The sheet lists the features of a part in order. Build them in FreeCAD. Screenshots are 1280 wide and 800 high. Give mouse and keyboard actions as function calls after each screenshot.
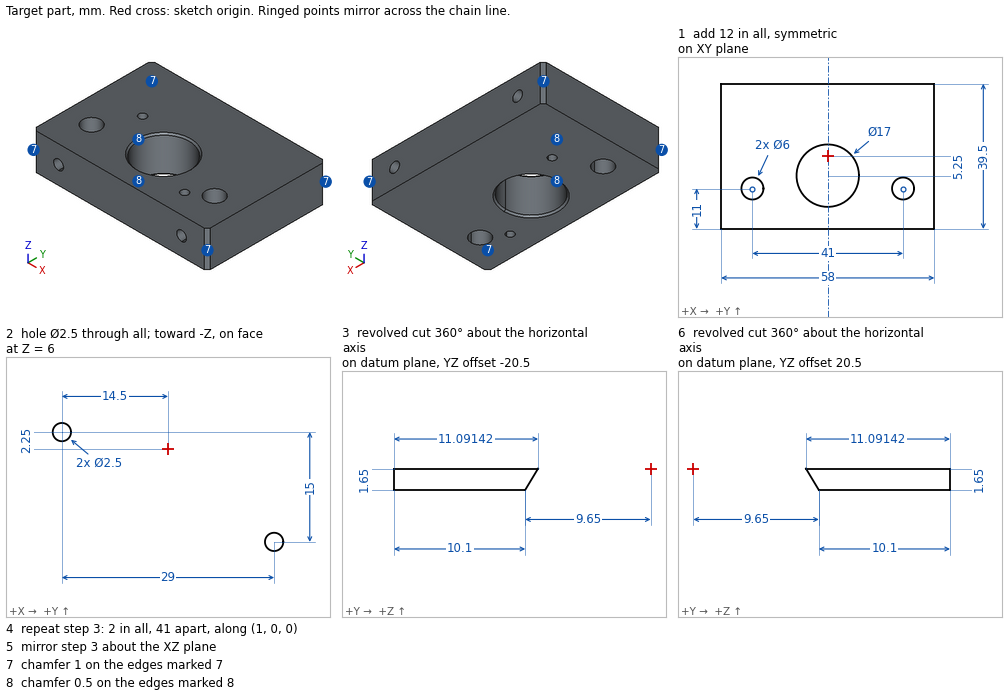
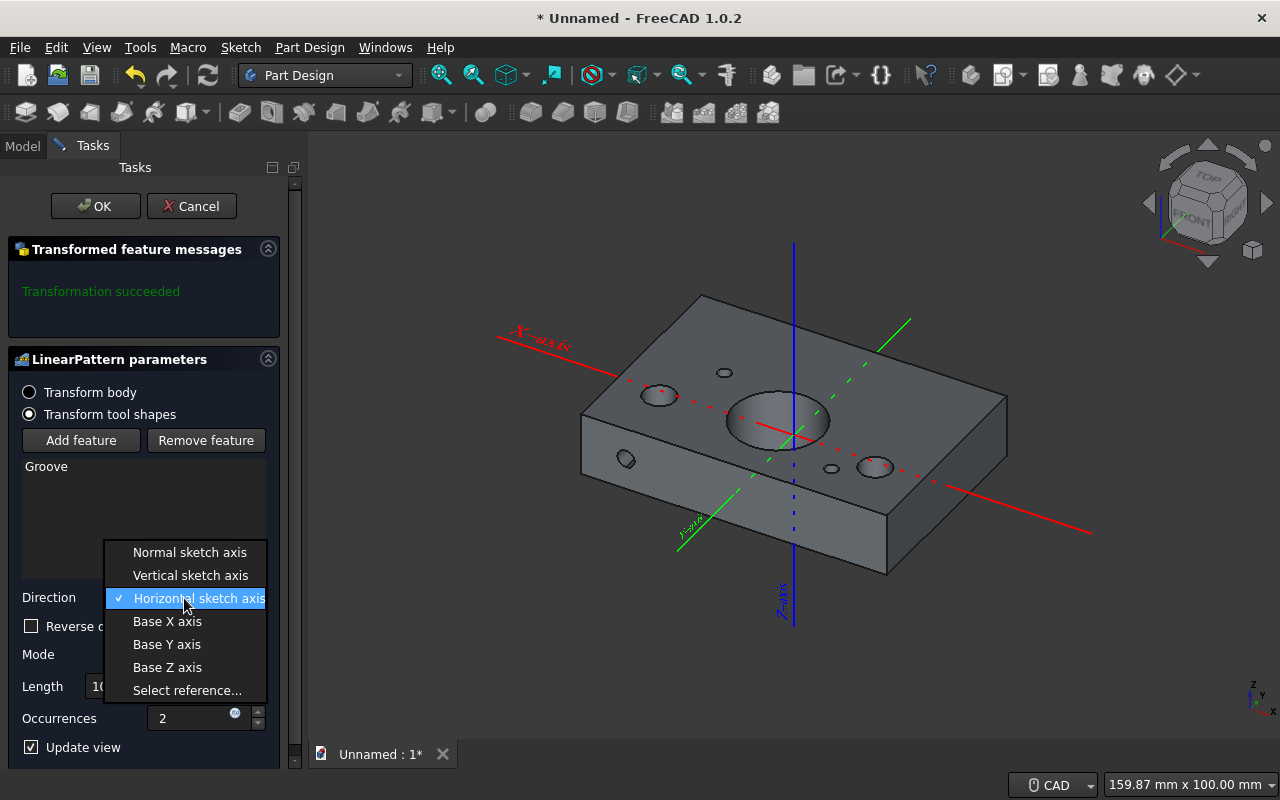
click(184, 622)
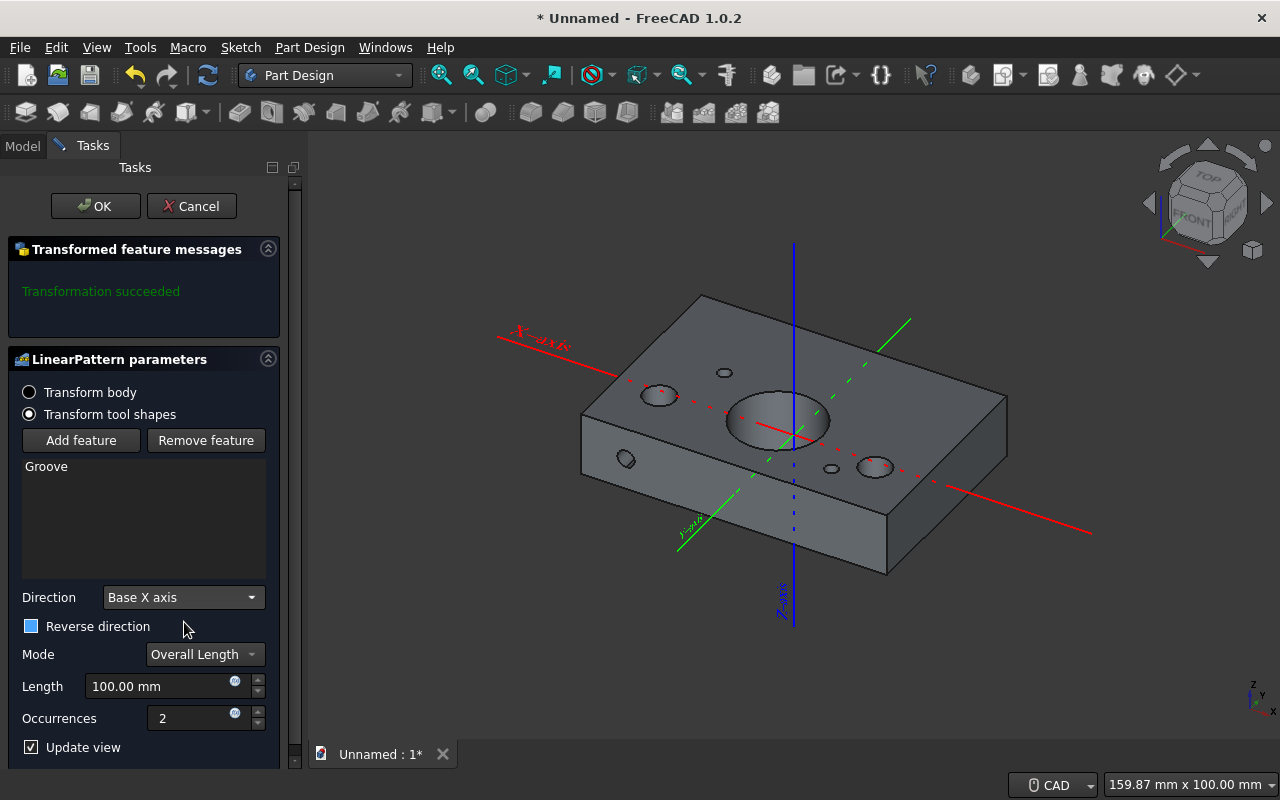
click(206, 654)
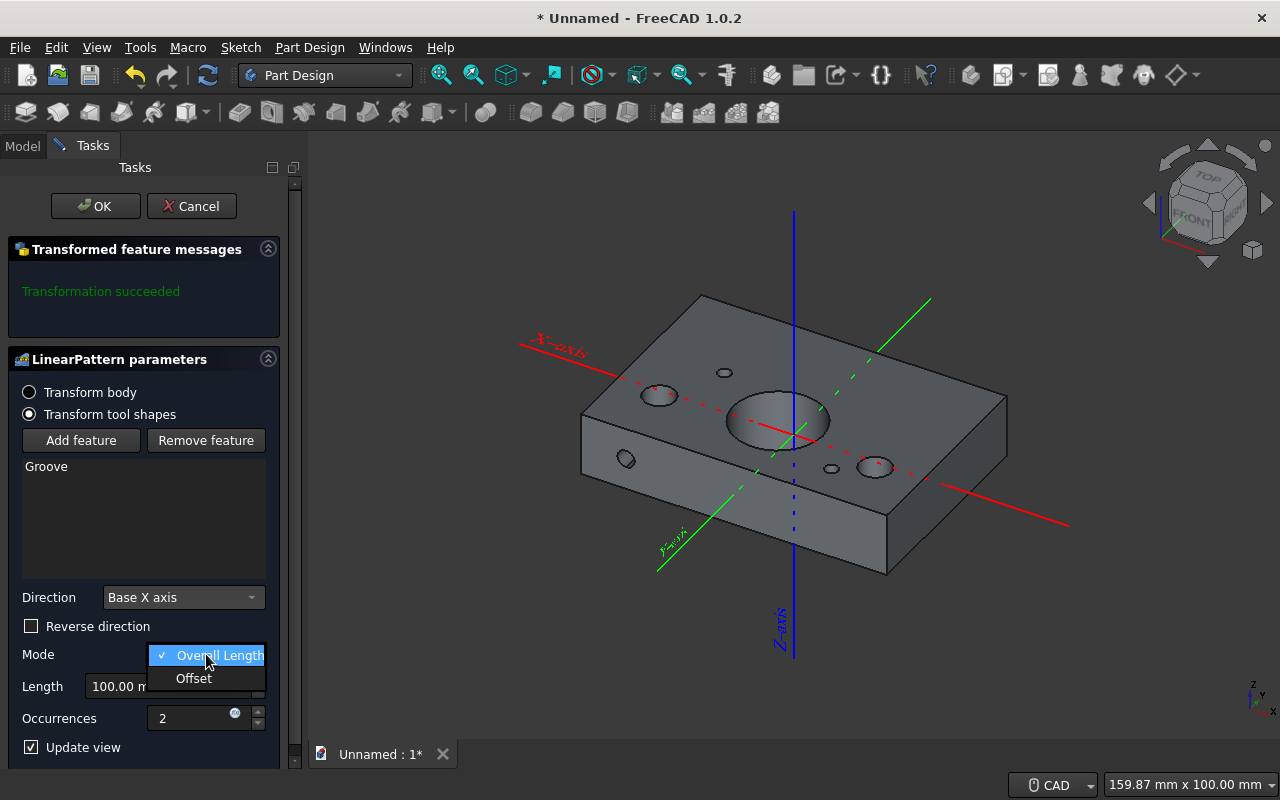
click(206, 678)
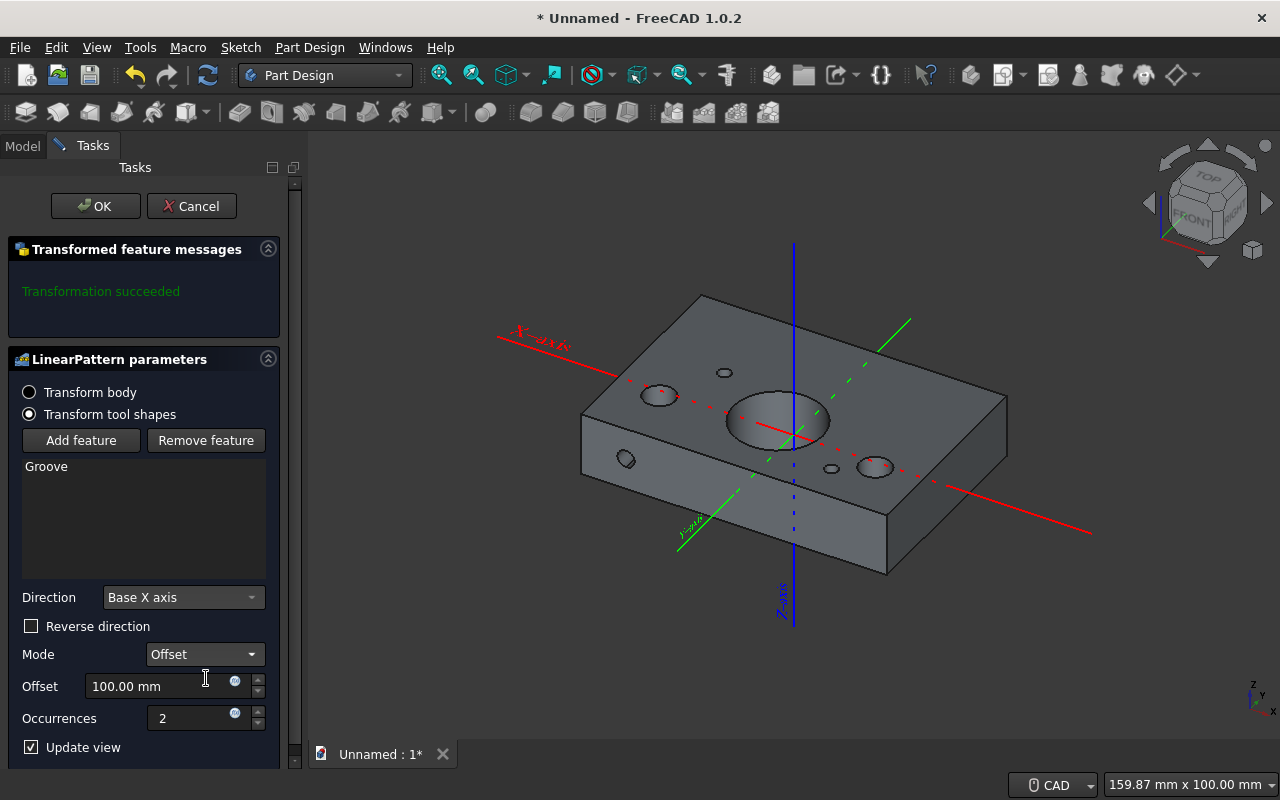
triple_click(168, 686)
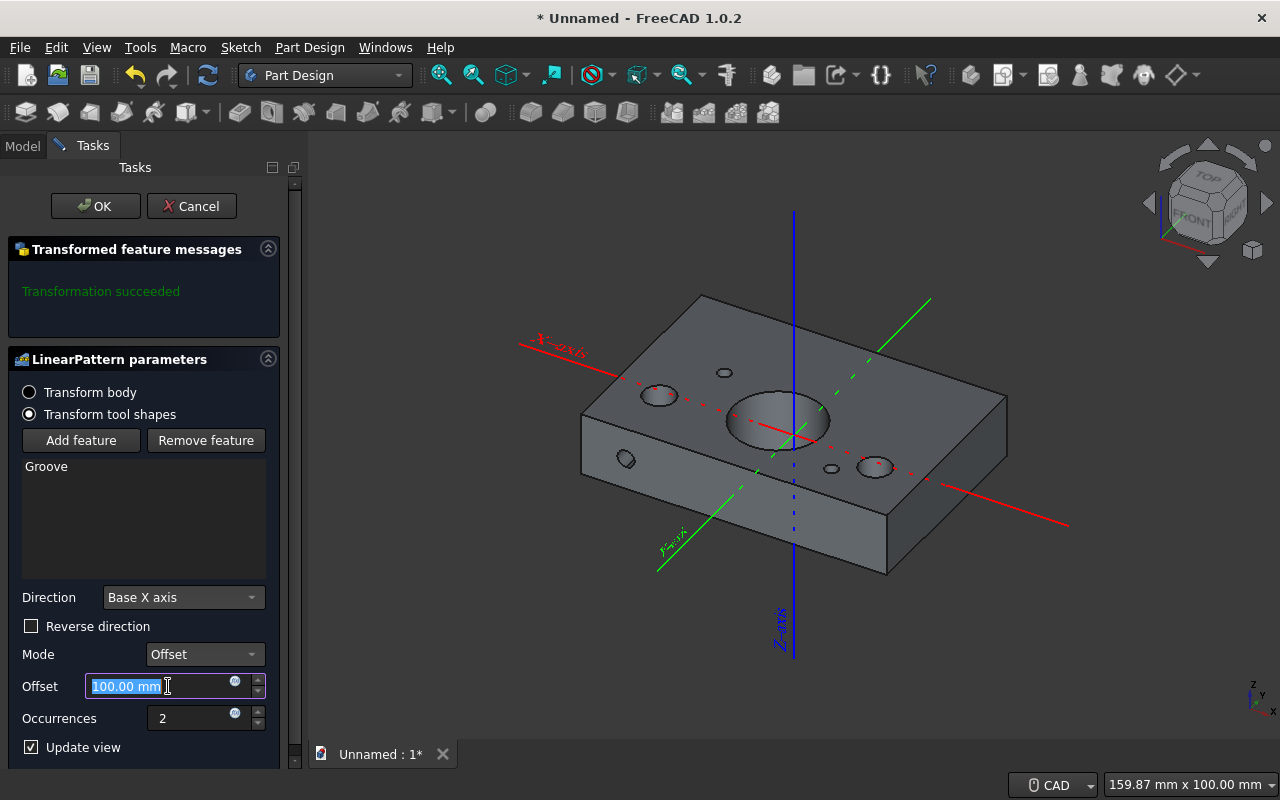
text(41)
key(Tab)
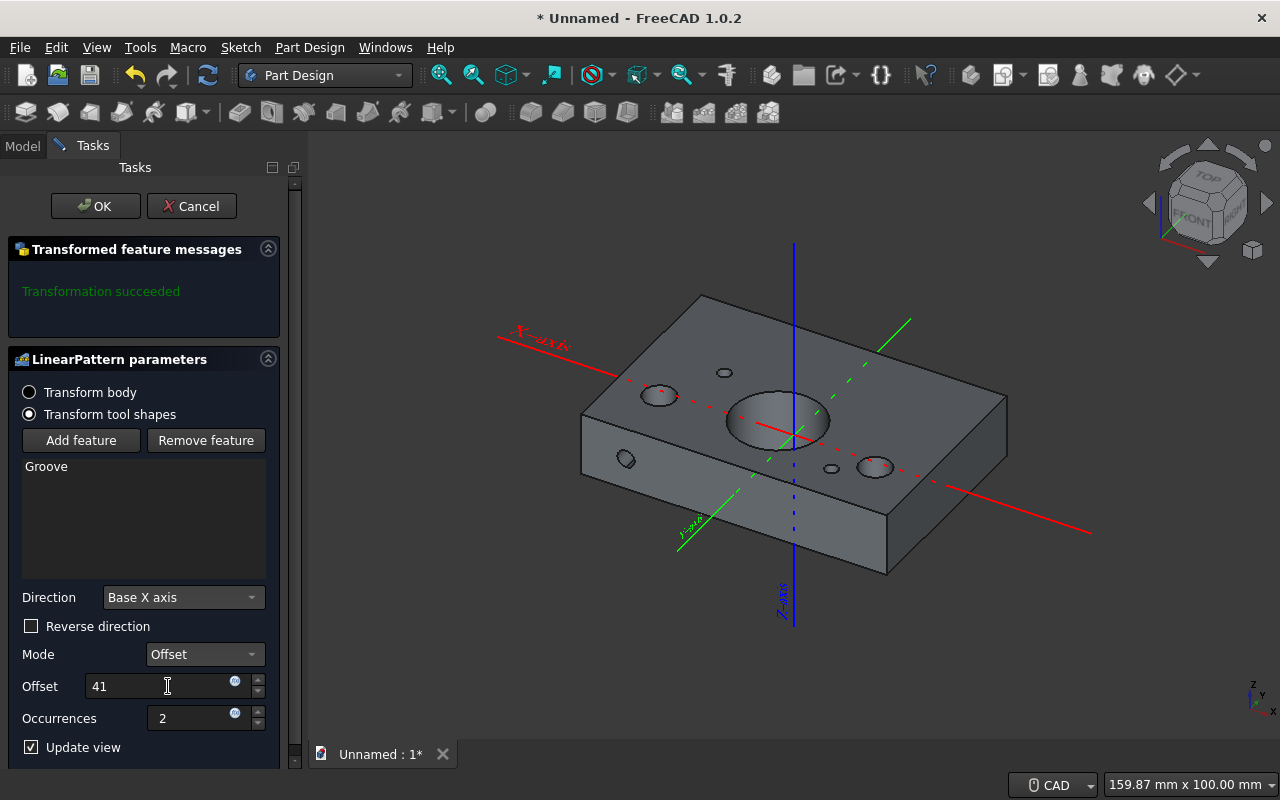
triple_click(198, 718)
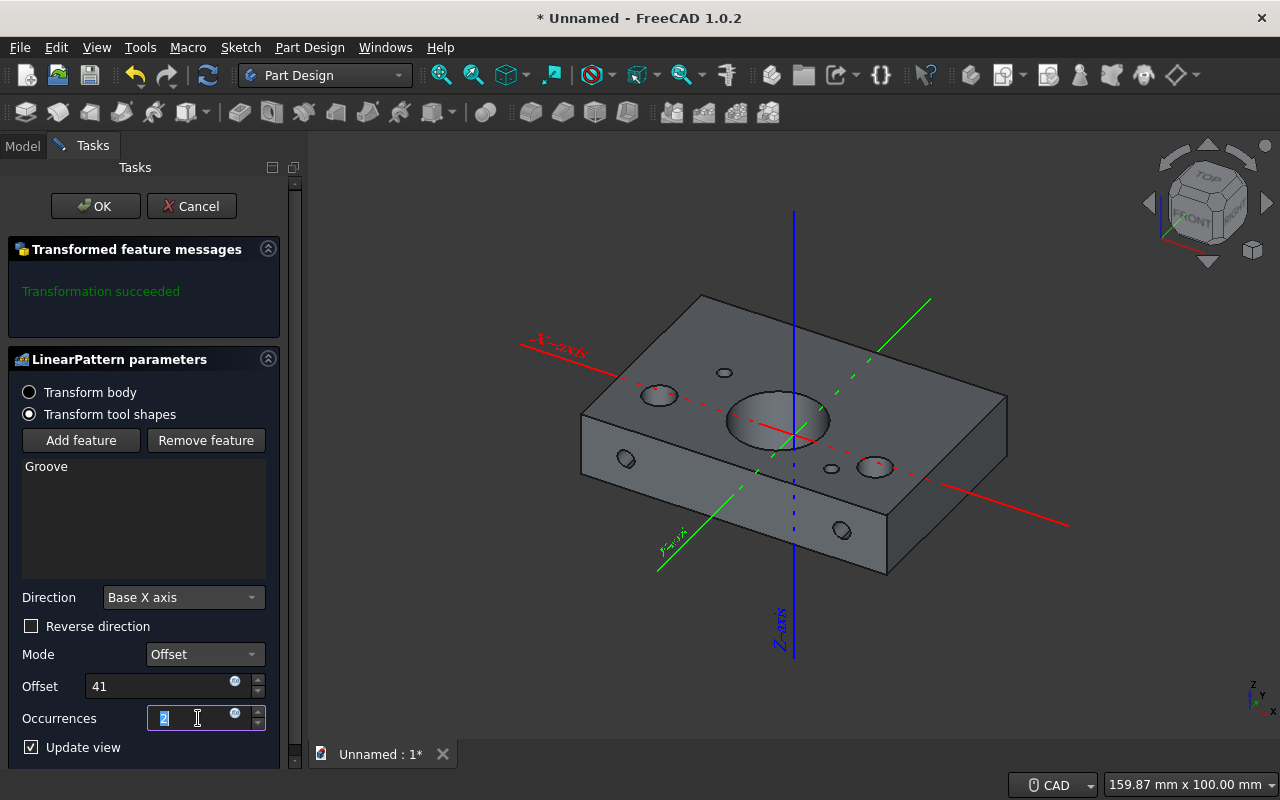
text(2)
key(Tab)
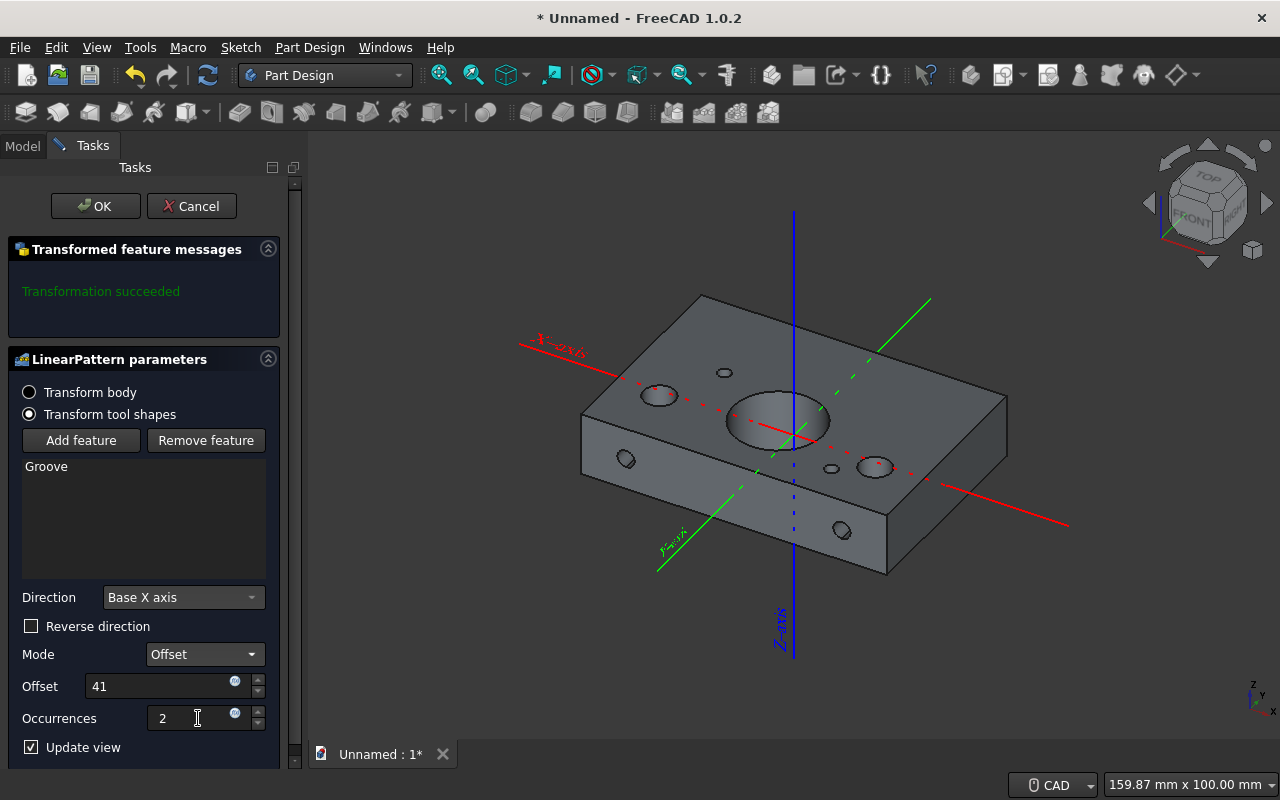
click(96, 206)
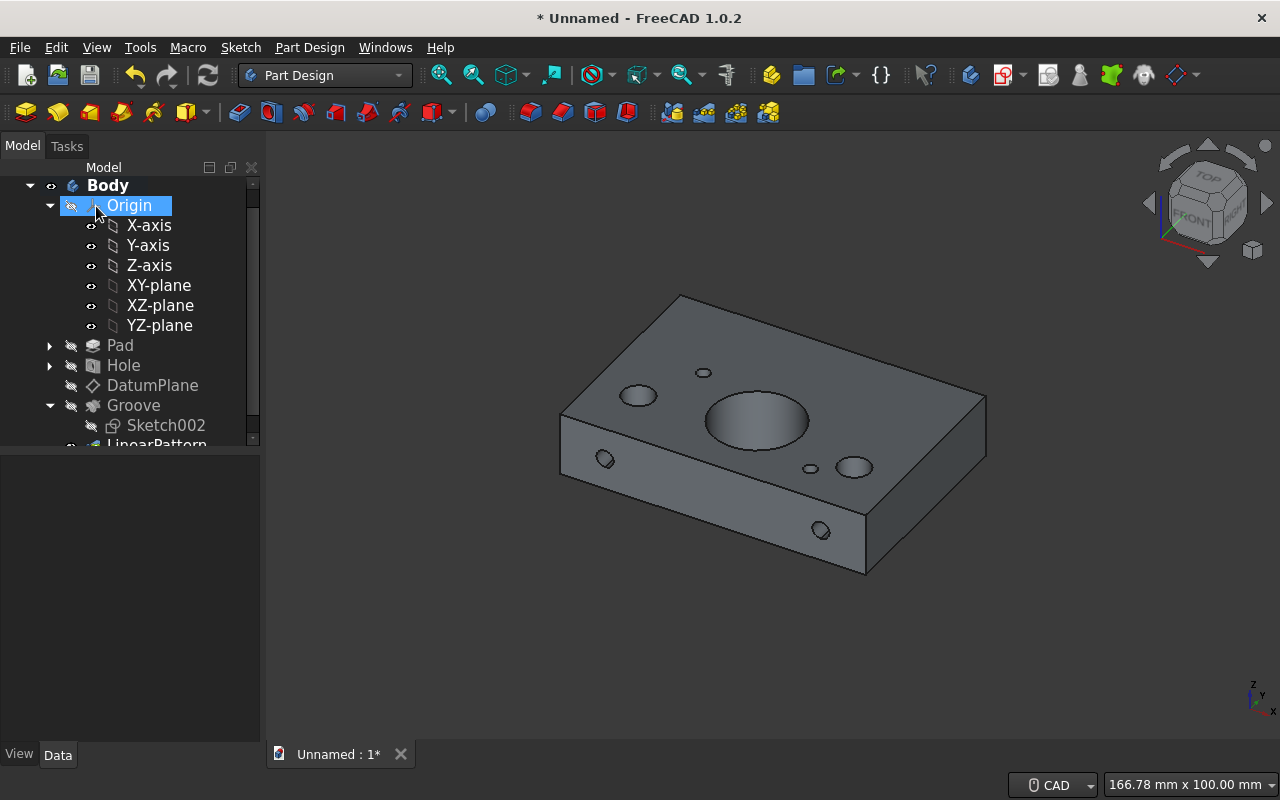
click(116, 406)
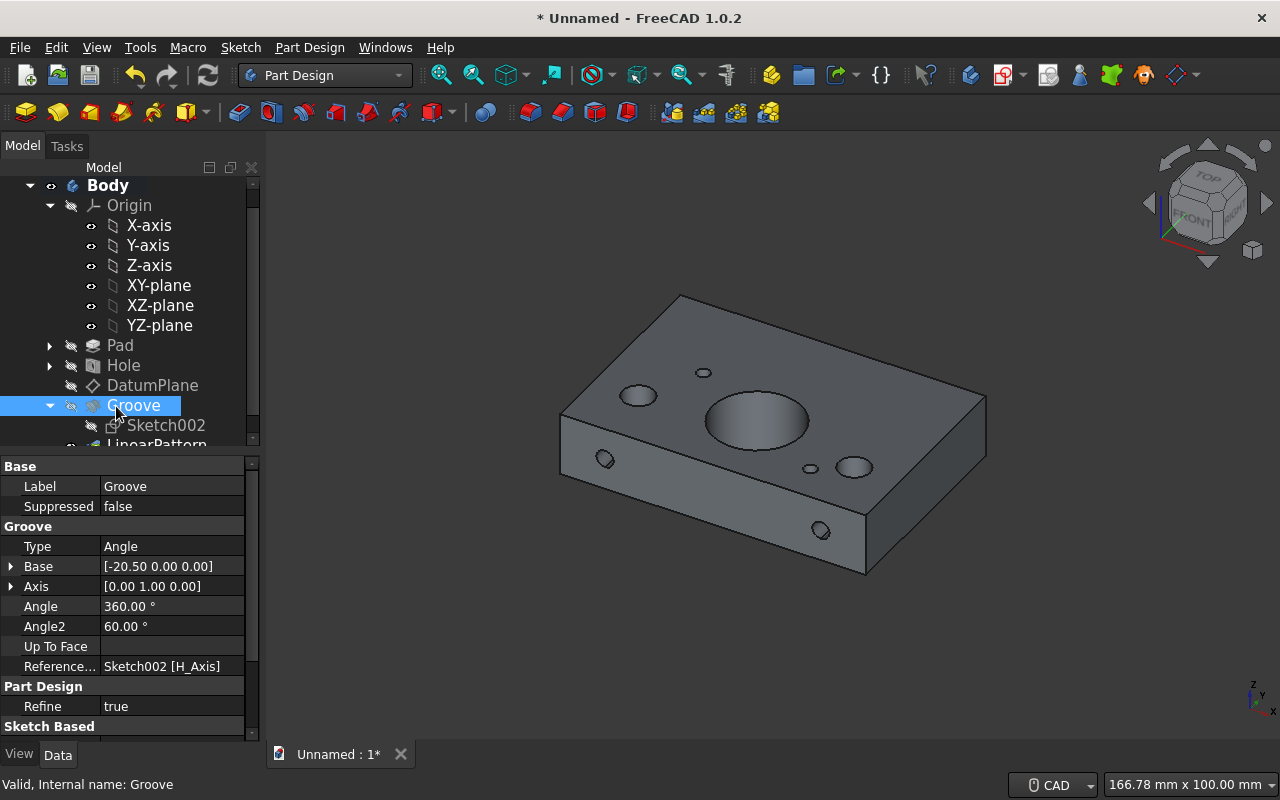
click(672, 112)